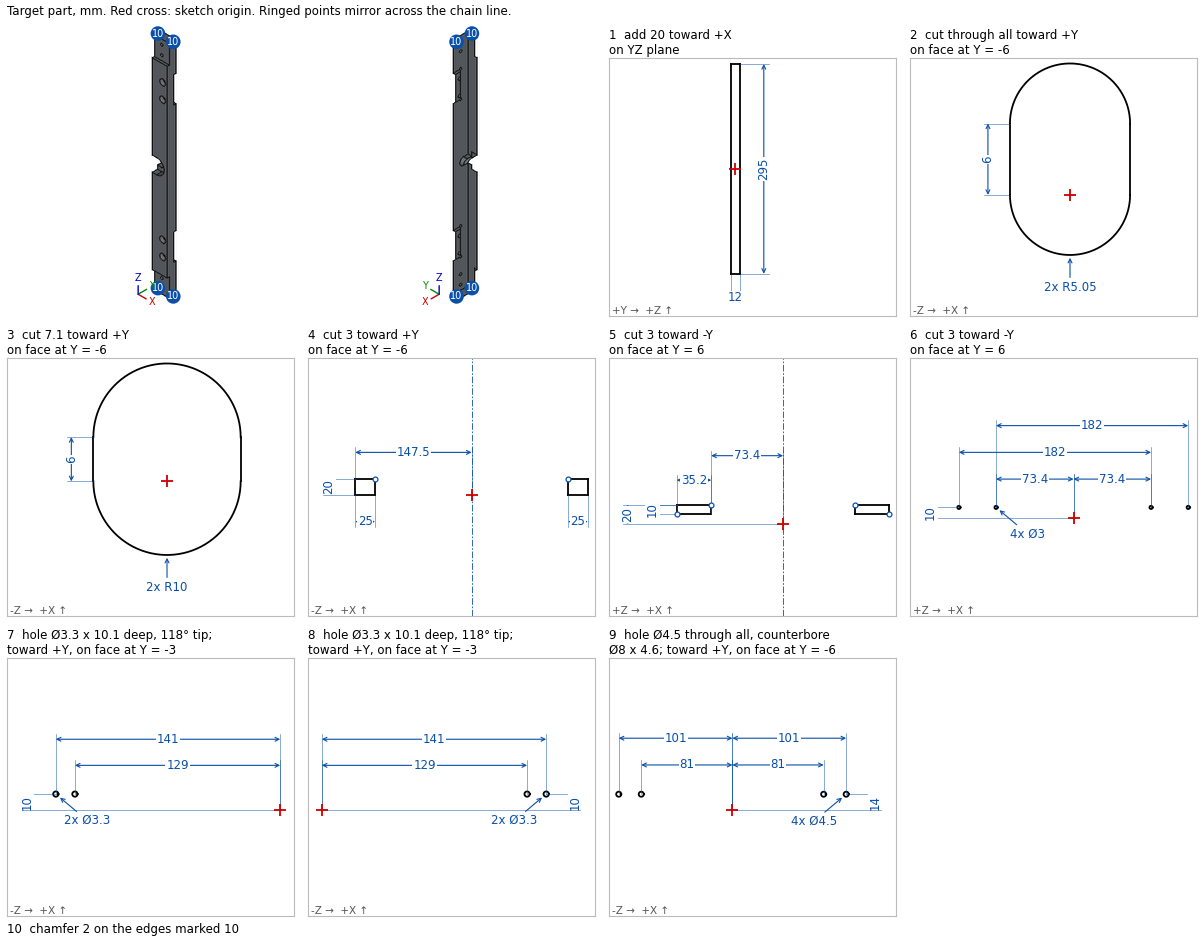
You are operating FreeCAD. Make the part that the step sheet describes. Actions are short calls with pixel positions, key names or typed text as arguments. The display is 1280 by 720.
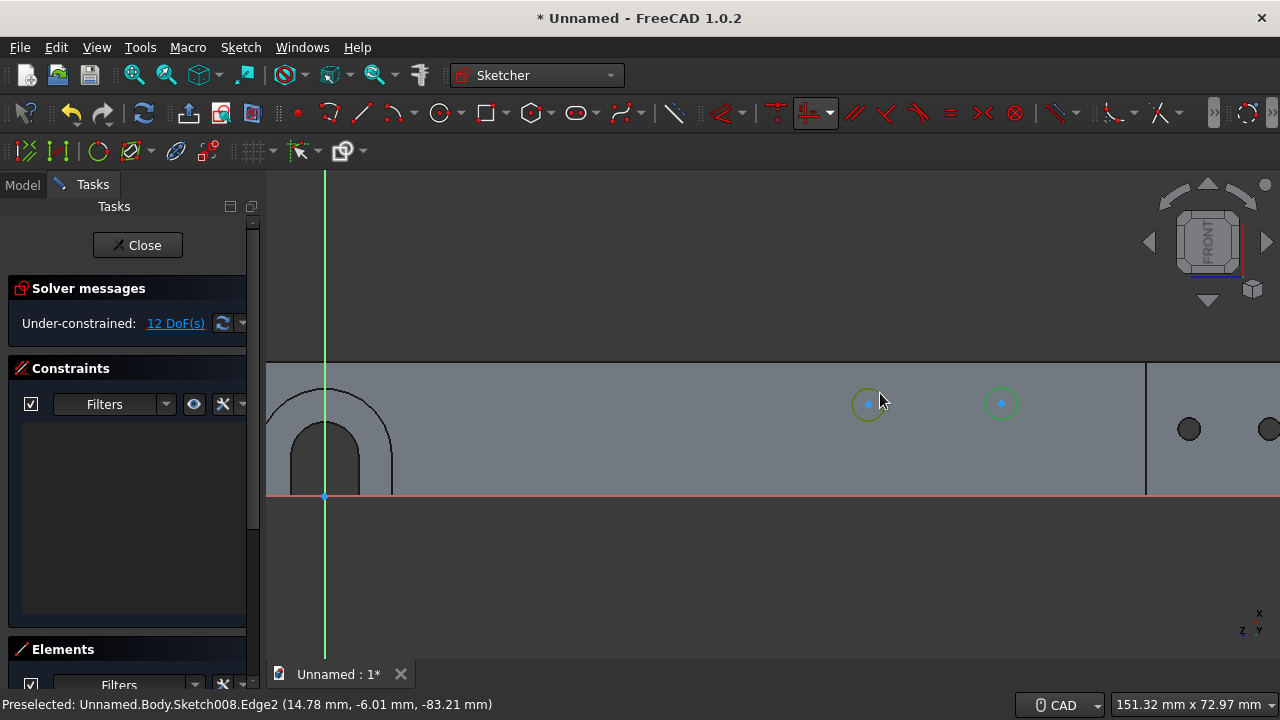
scroll(1014, 392, down, 4)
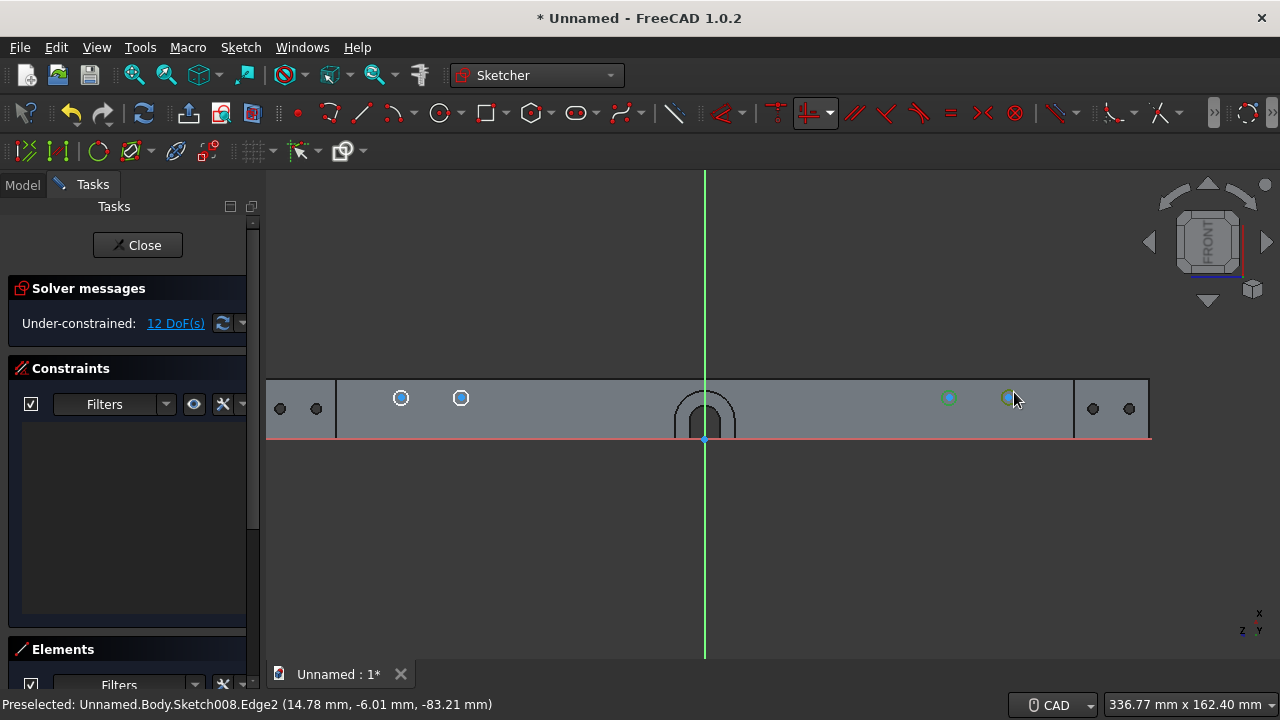
scroll(466, 393, up, 4)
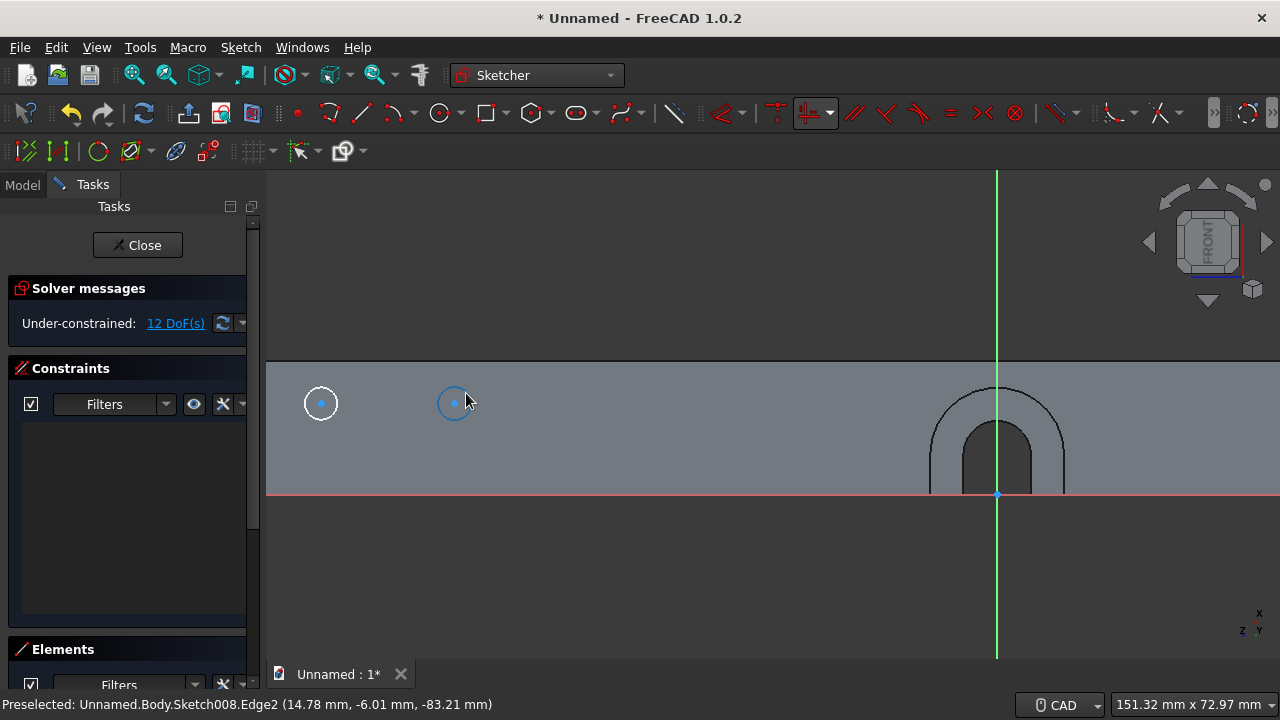
click(466, 392)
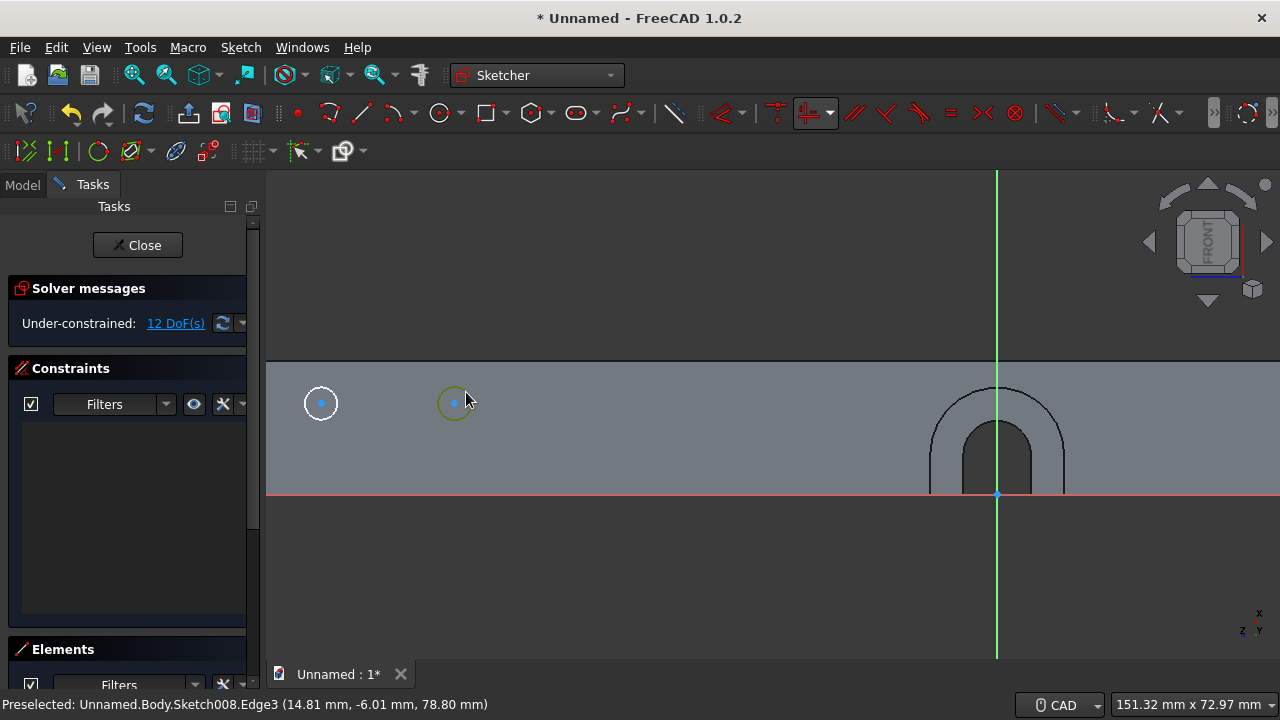
click(332, 392)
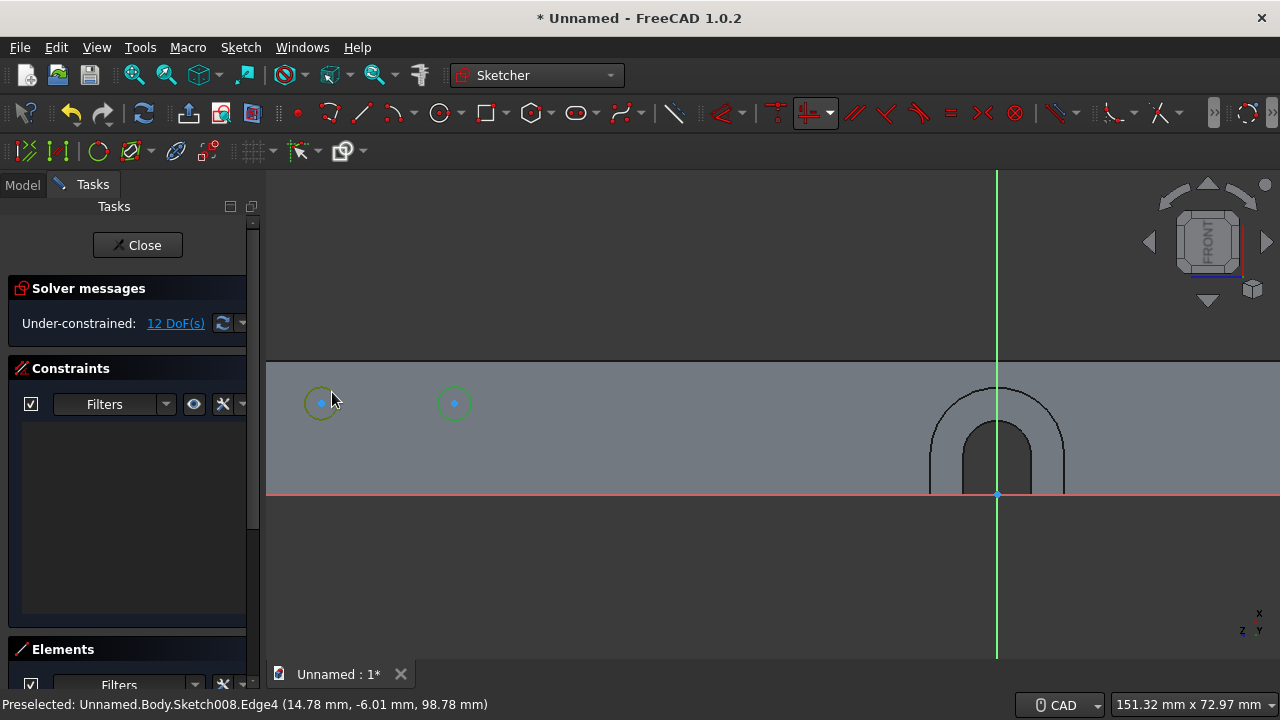
click(952, 114)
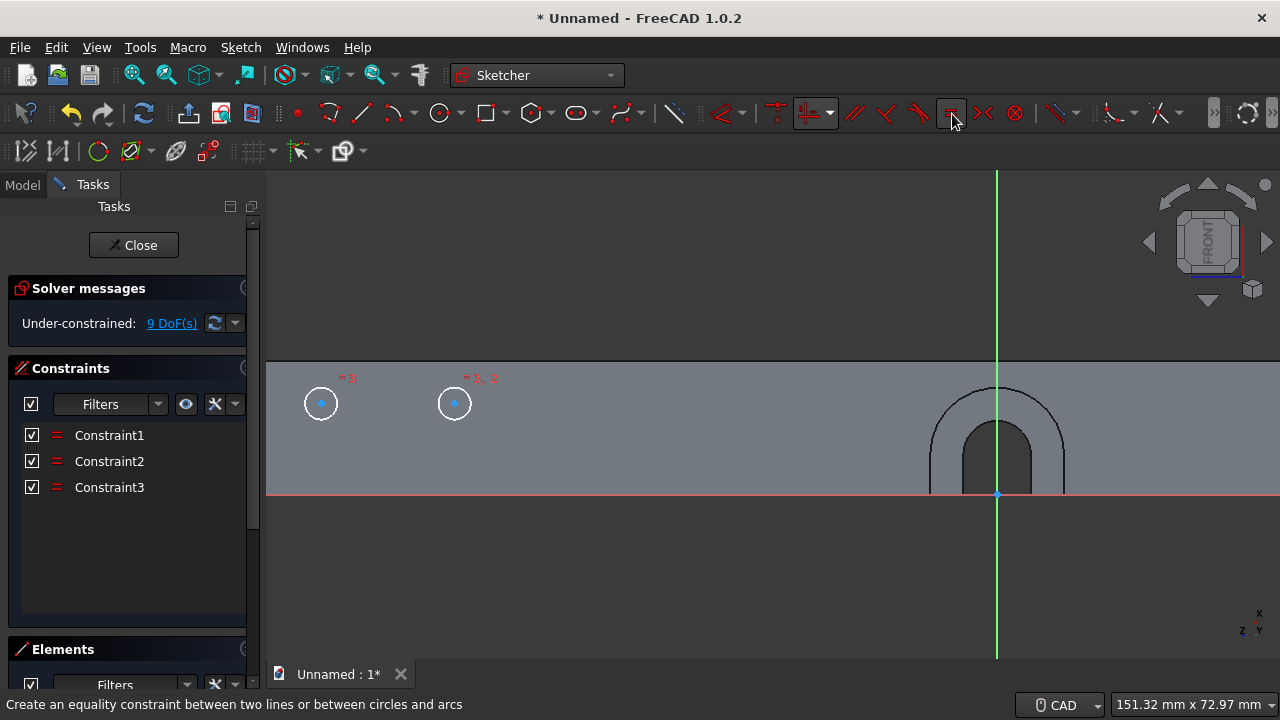
scroll(466, 393, down, 4)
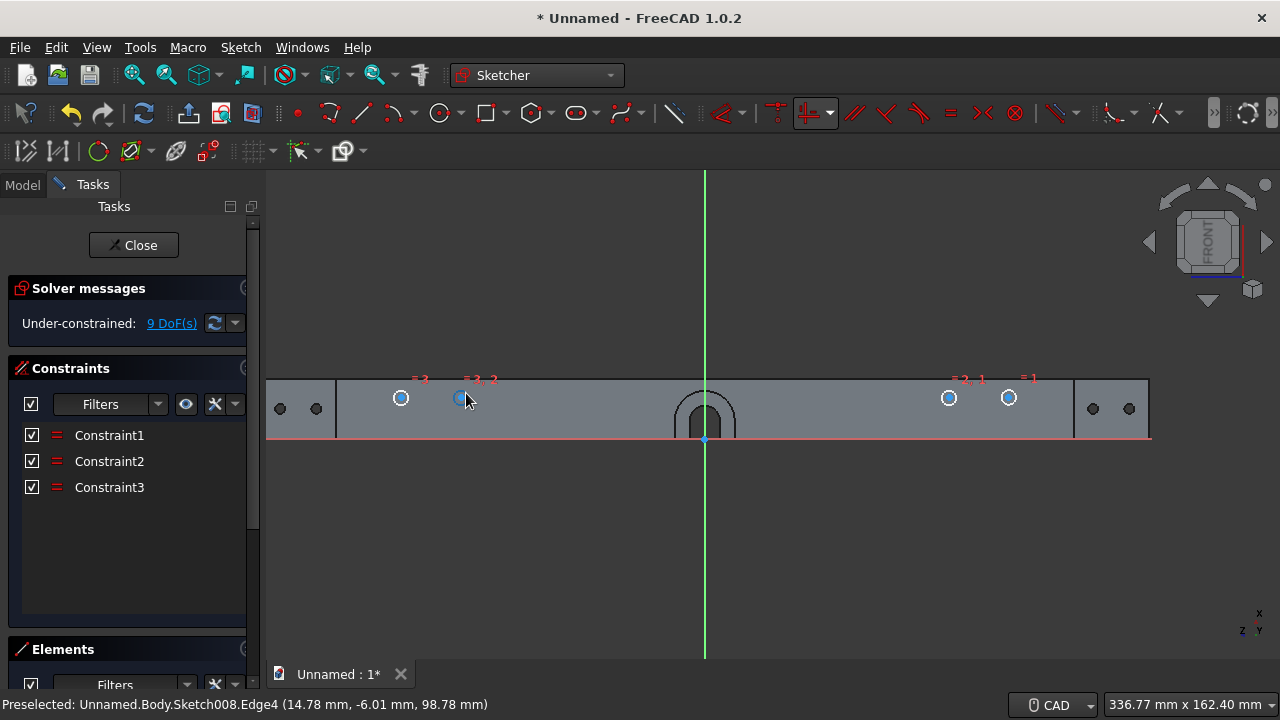
click(1009, 397)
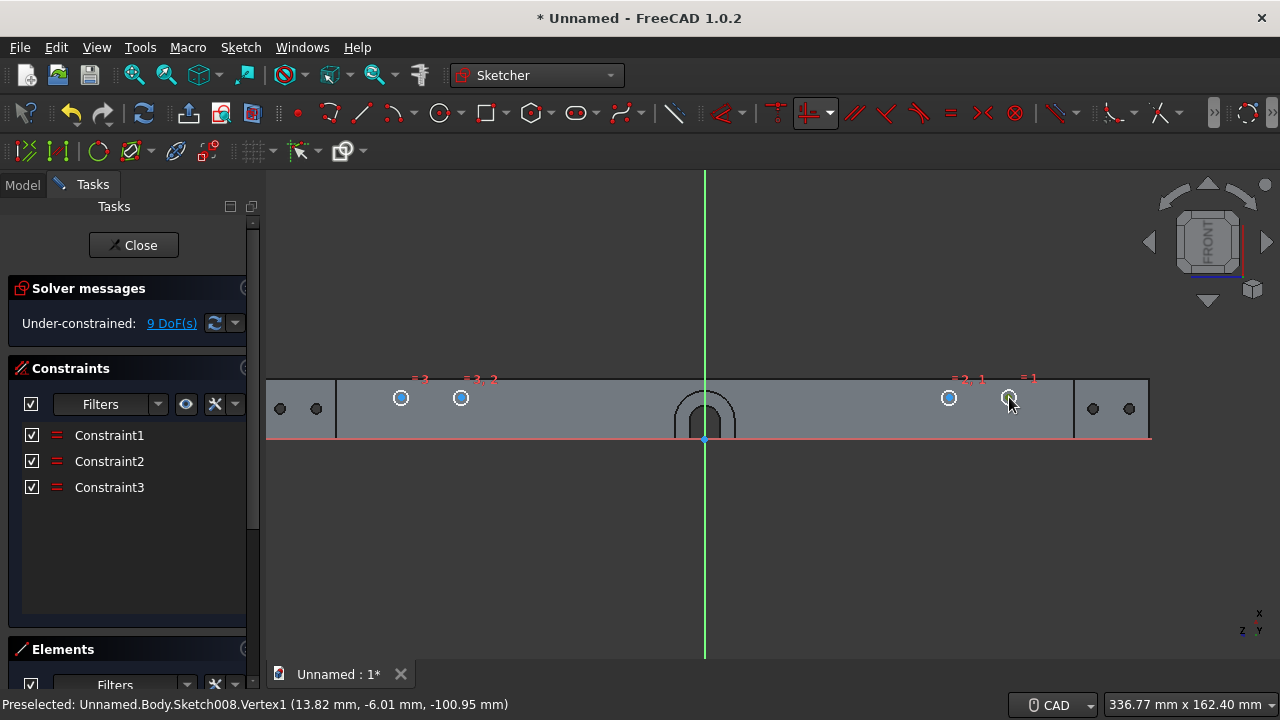
click(949, 398)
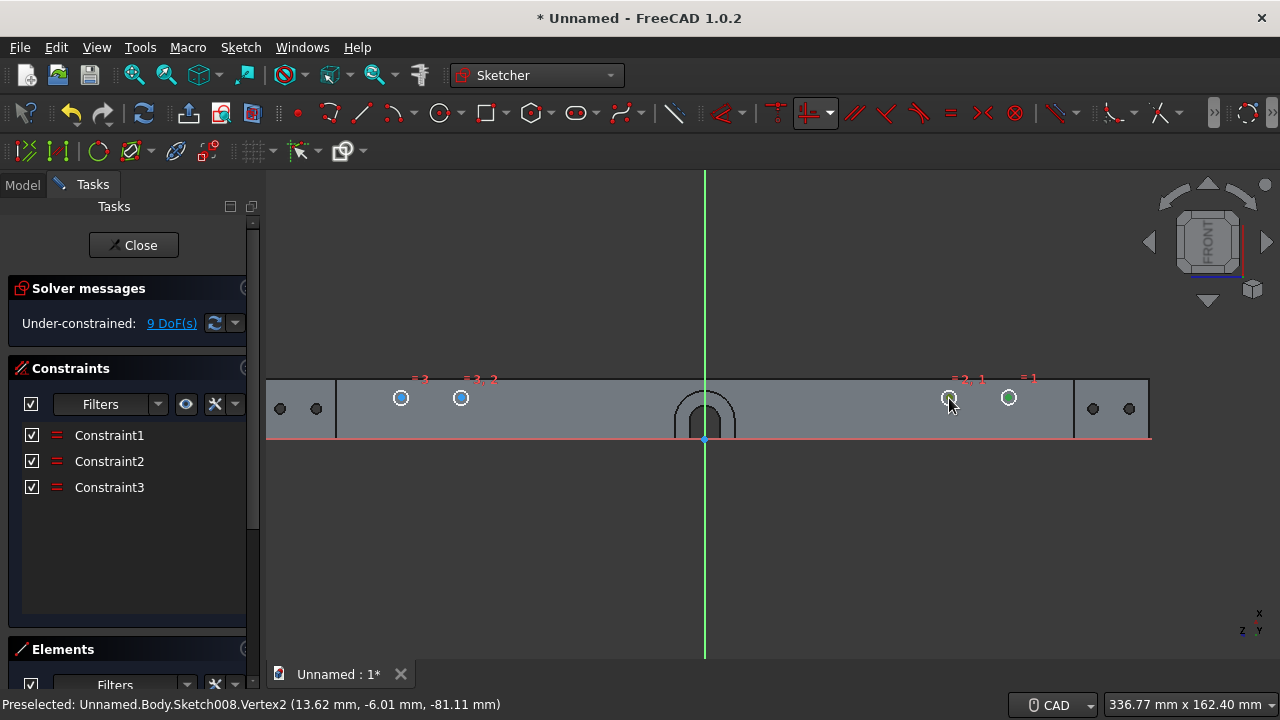
click(832, 114)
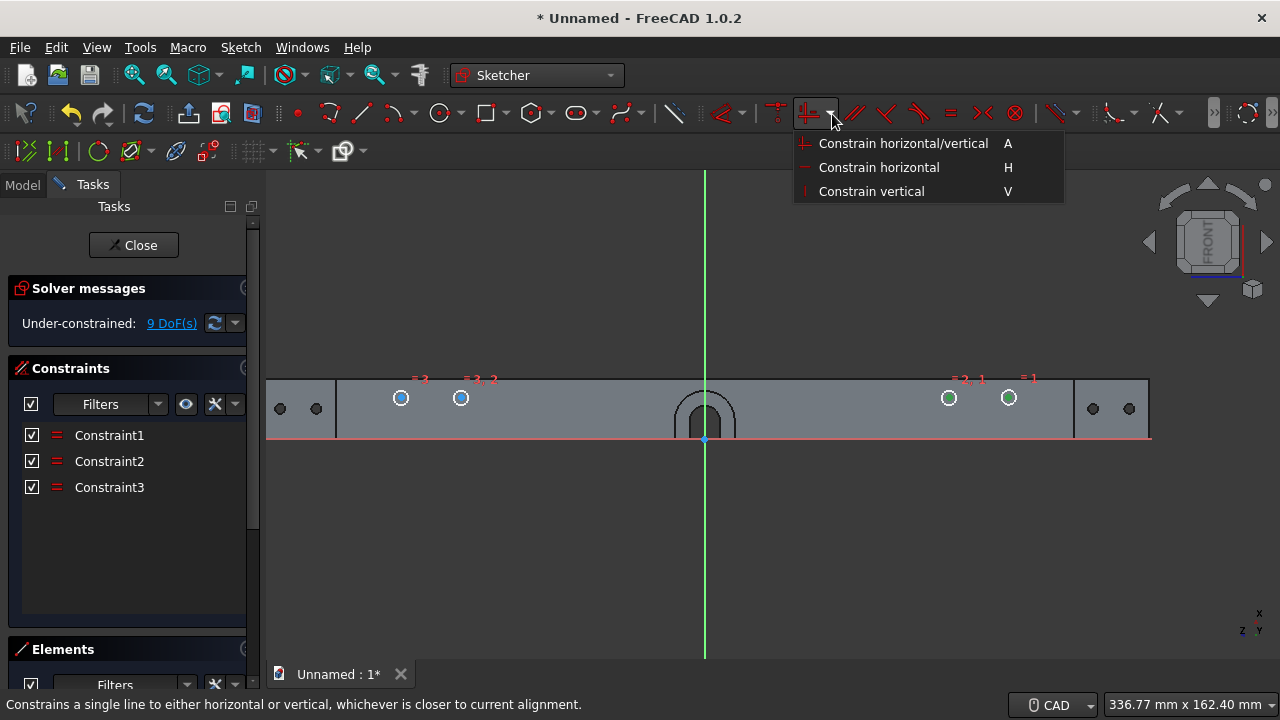
click(929, 167)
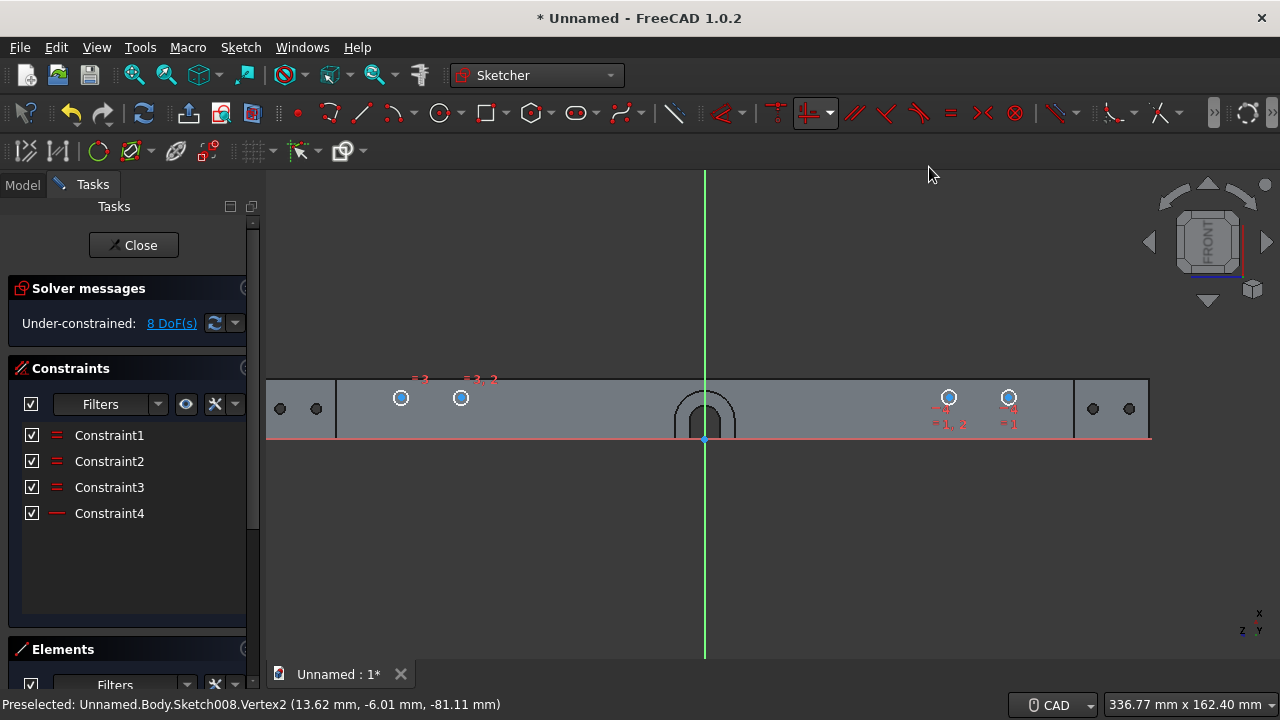
click(949, 397)